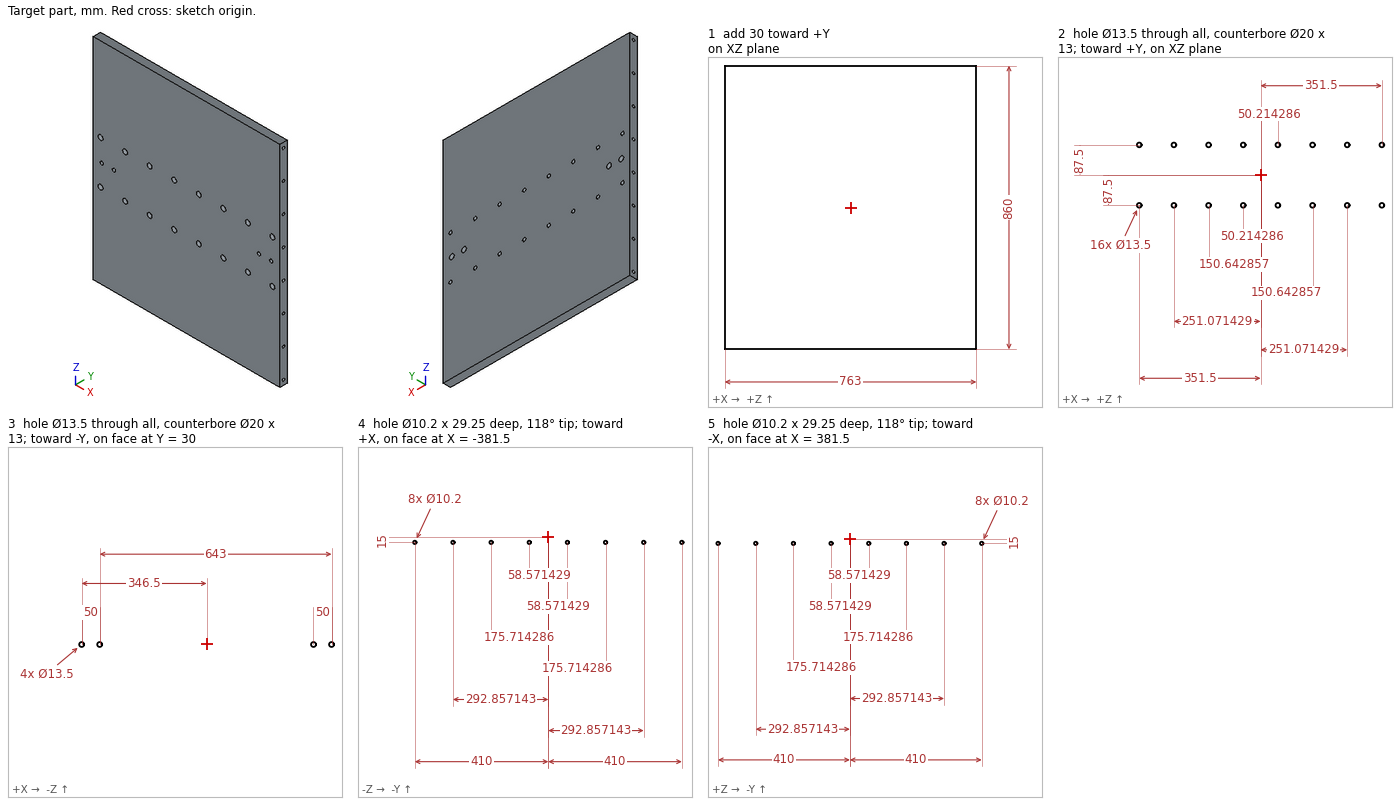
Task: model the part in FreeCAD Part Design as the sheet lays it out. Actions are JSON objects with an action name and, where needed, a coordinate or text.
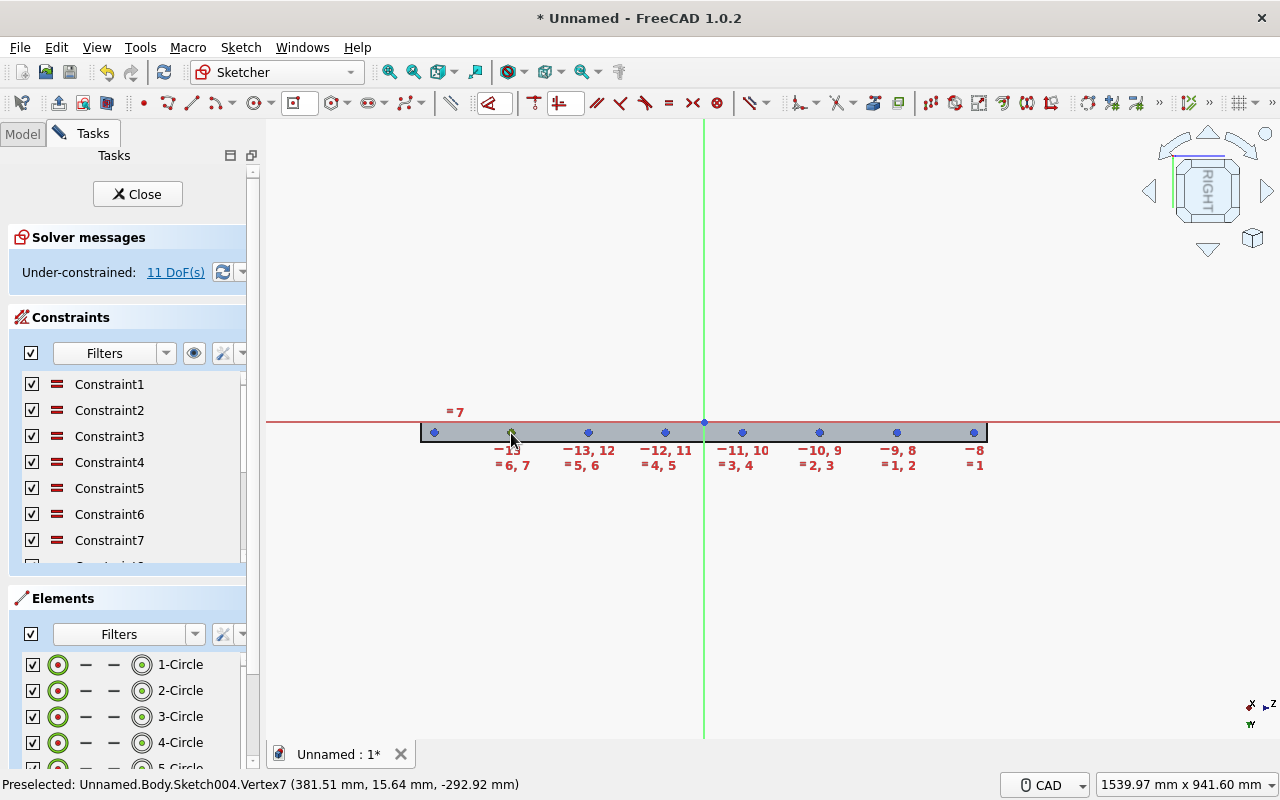
{"action": "left_click", "coordinate": [434, 433]}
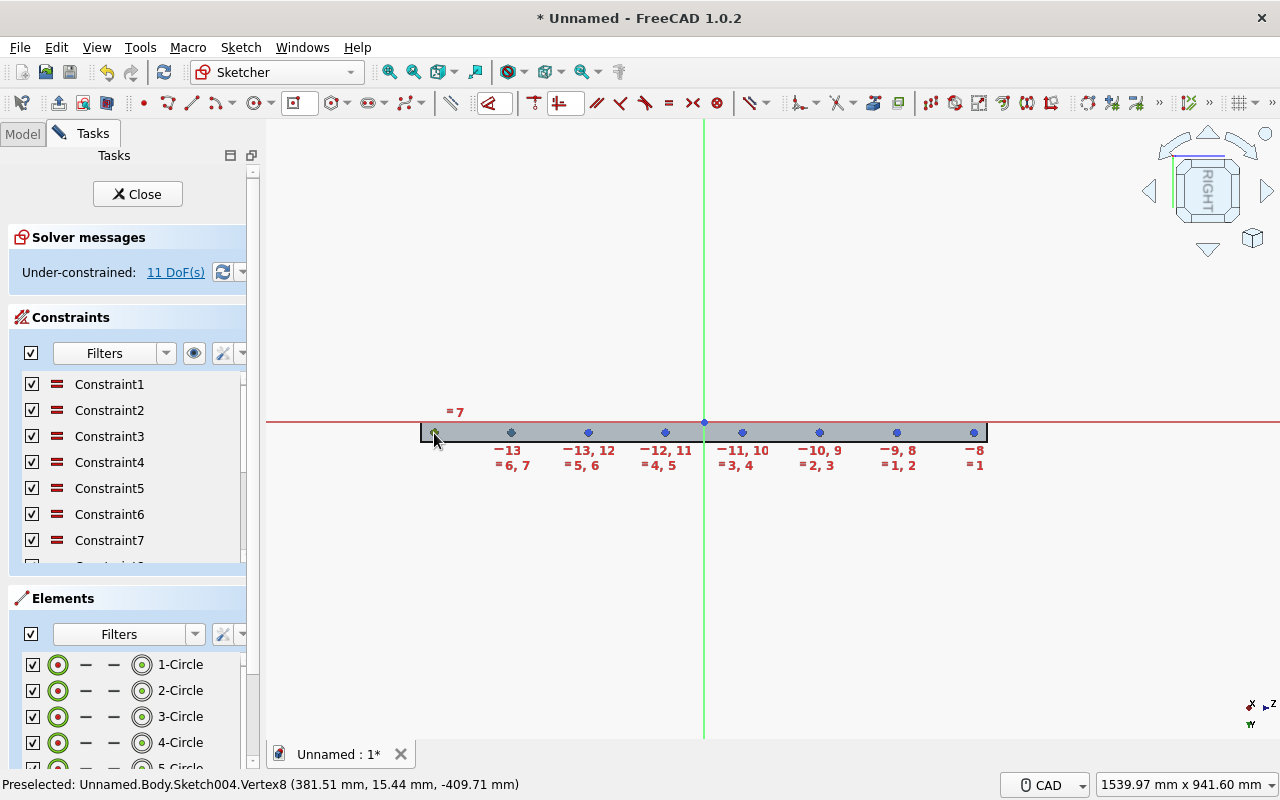
{"action": "key", "text": "h"}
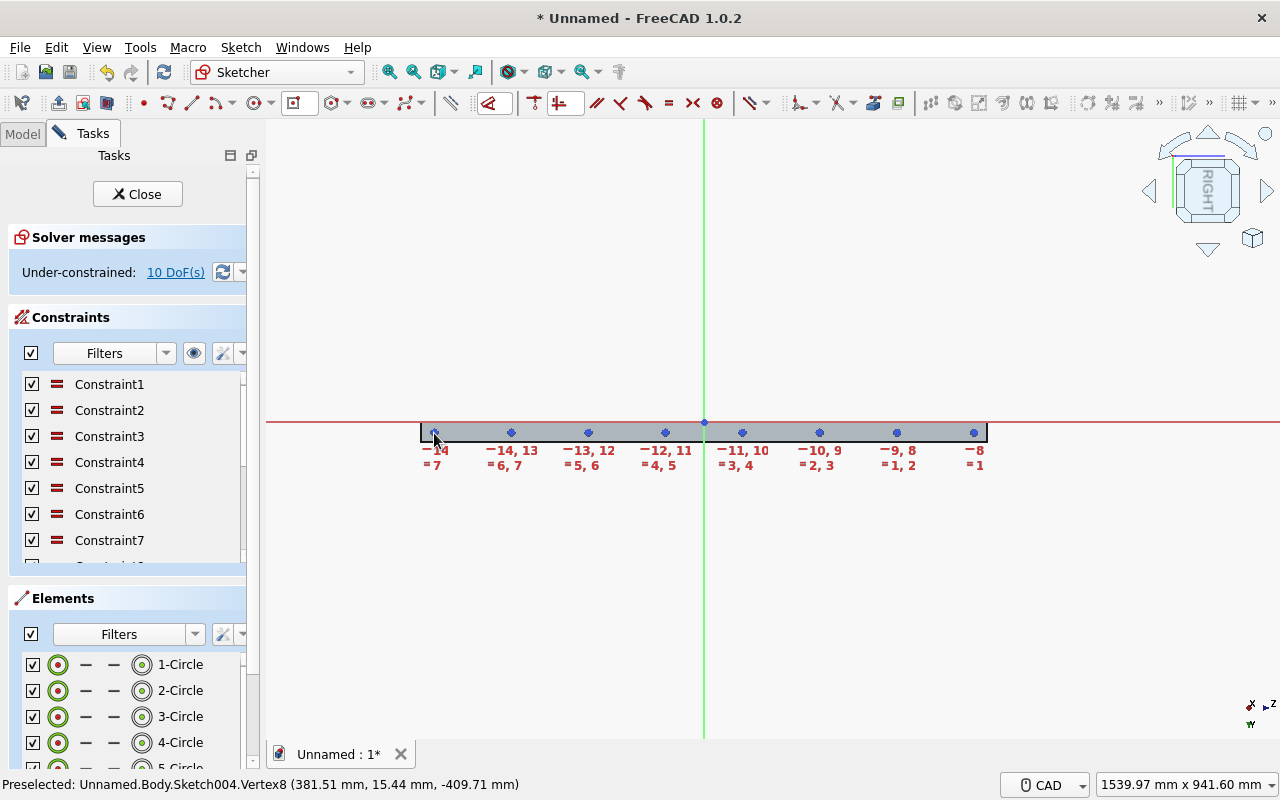
{"action": "scroll", "coordinate": [976, 435], "scroll_direction": "up", "scroll_amount": 9}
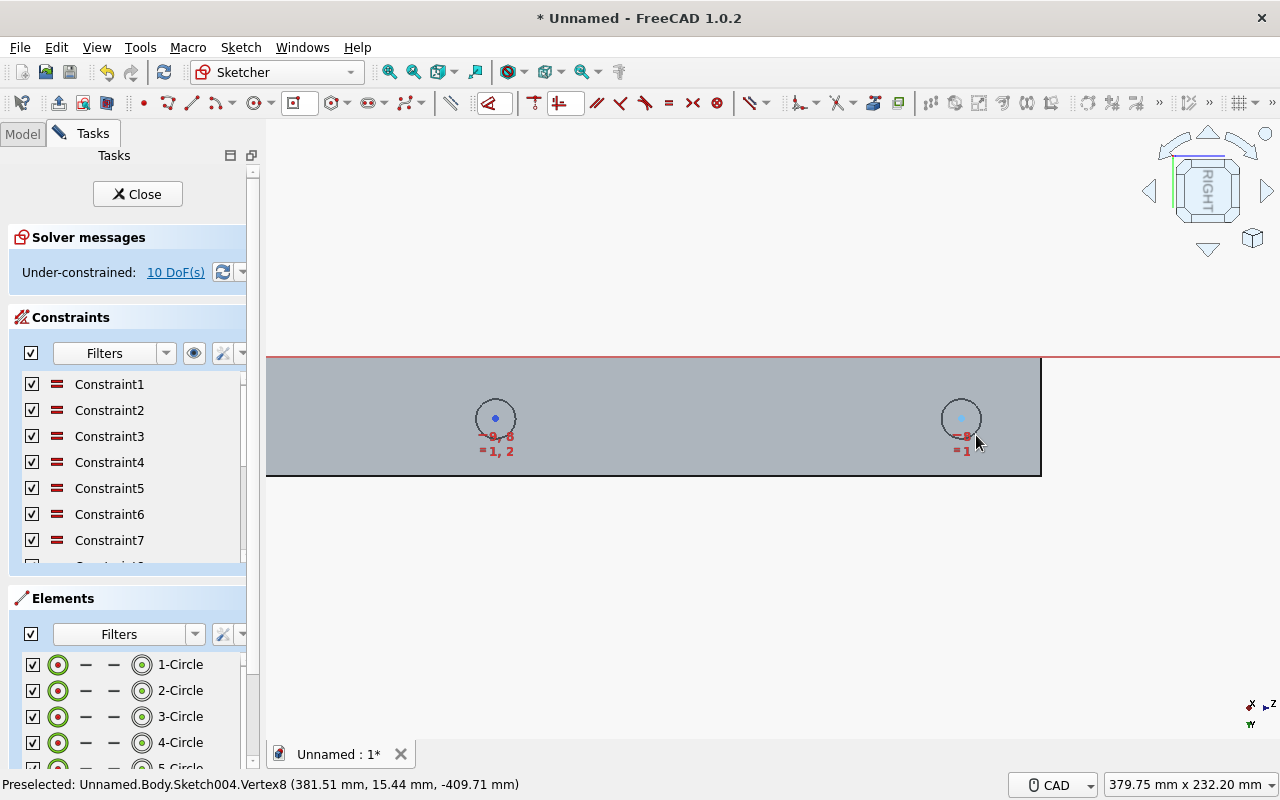
{"action": "left_click", "coordinate": [975, 433]}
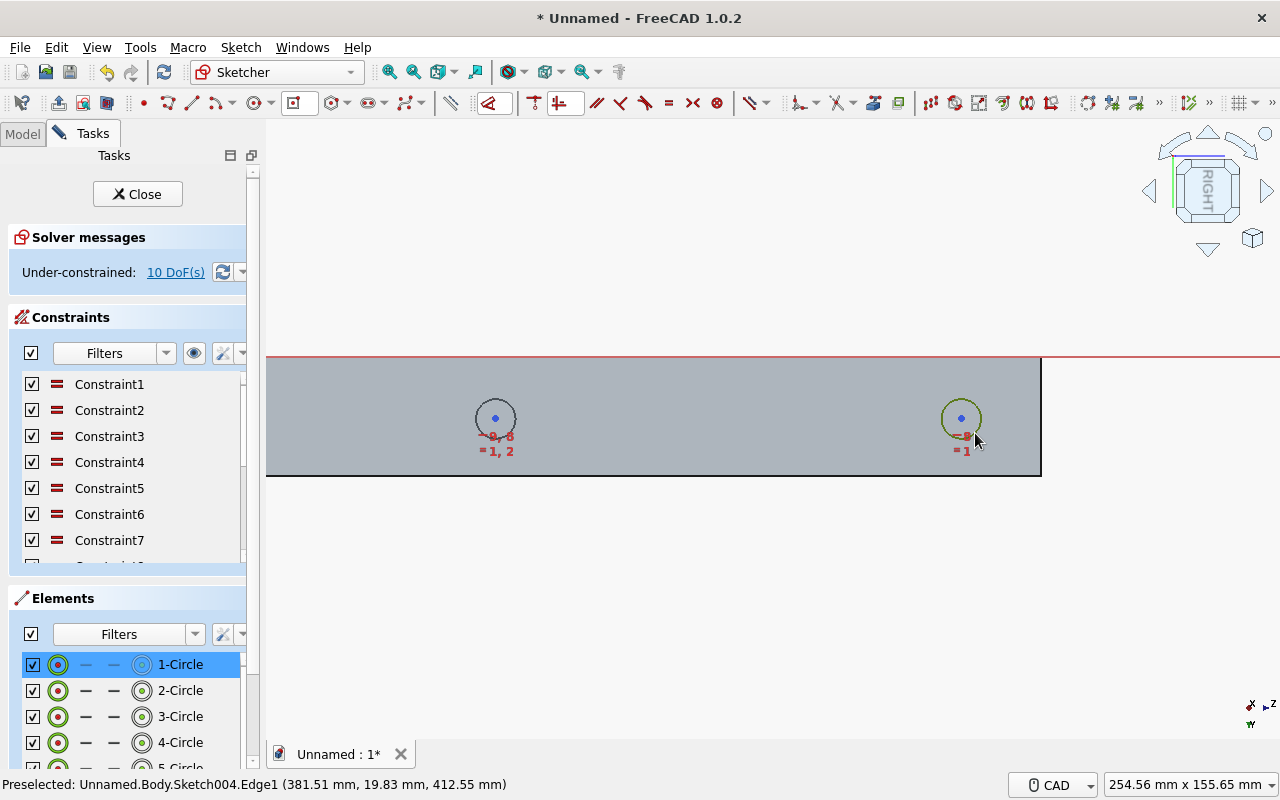
{"action": "key", "text": "k o"}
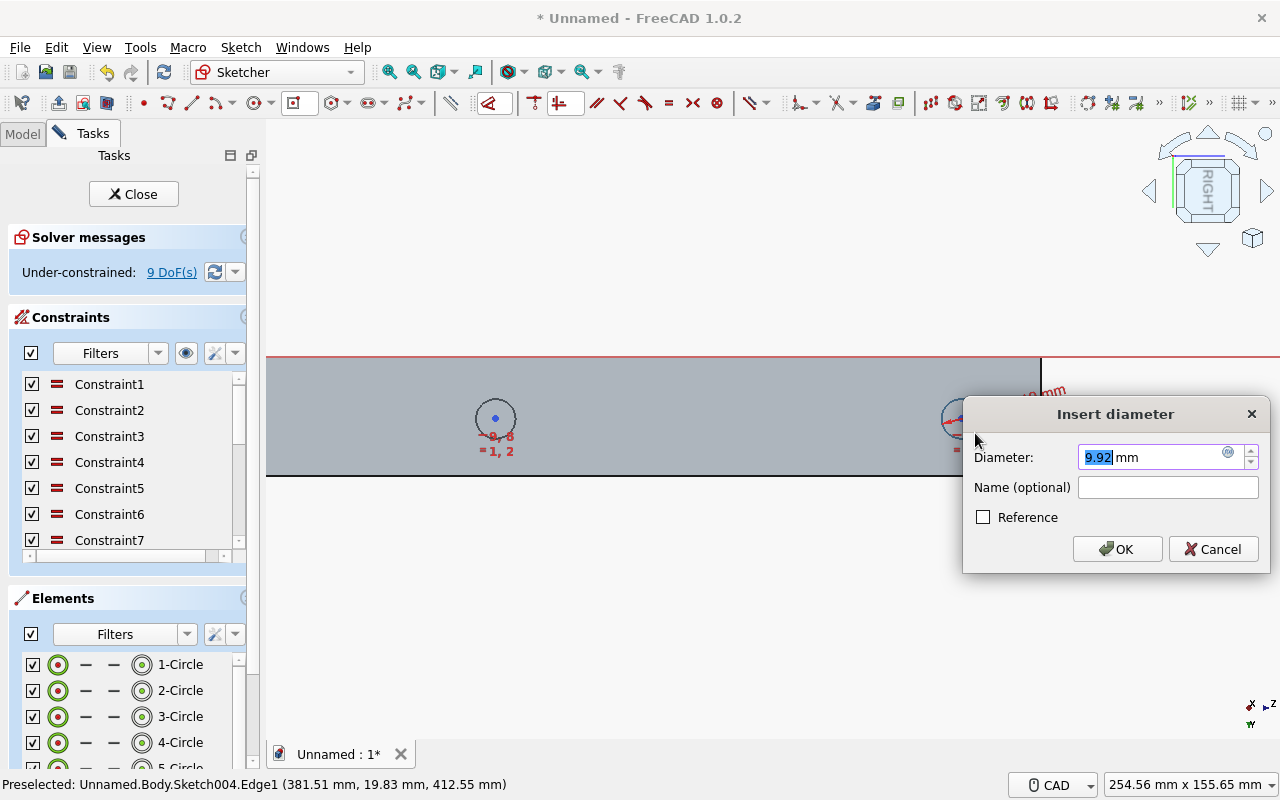
{"action": "type", "text": "10.2"}
{"action": "key", "text": "Return"}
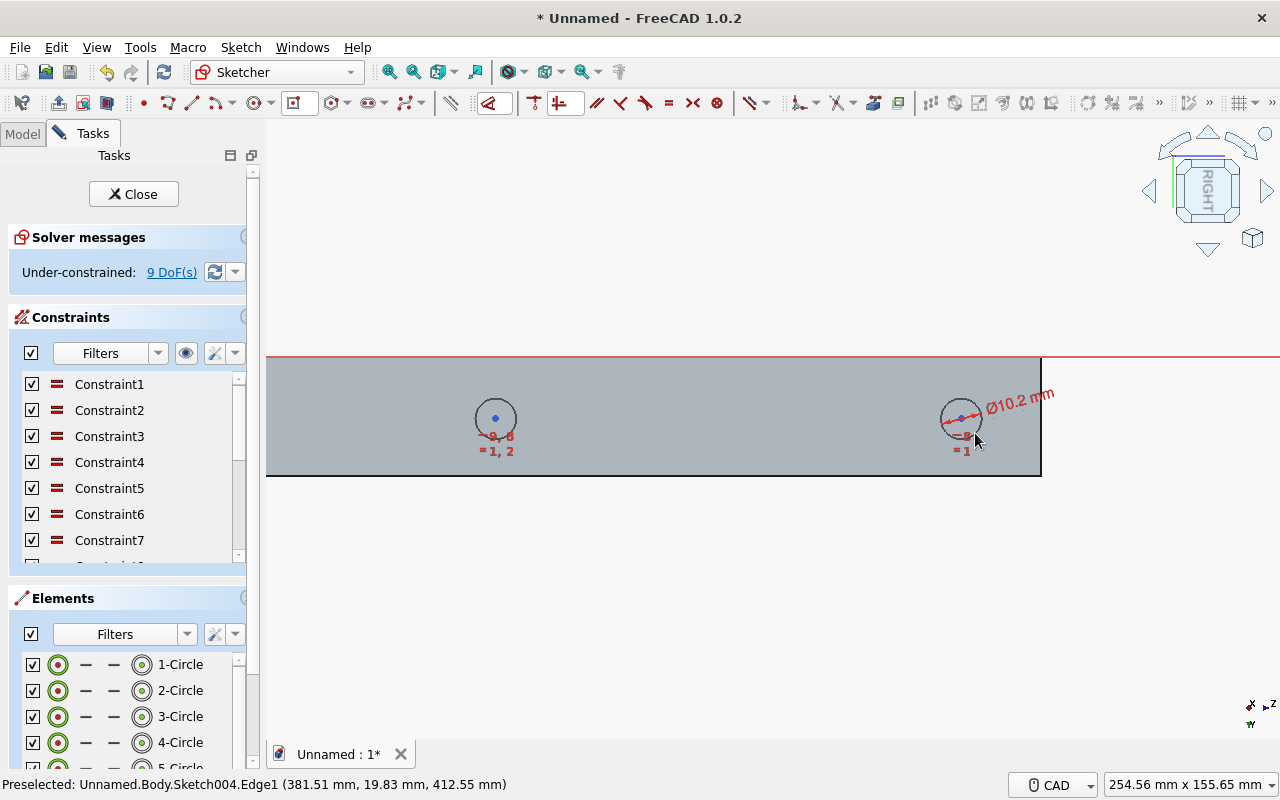
{"action": "left_click", "coordinate": [961, 419]}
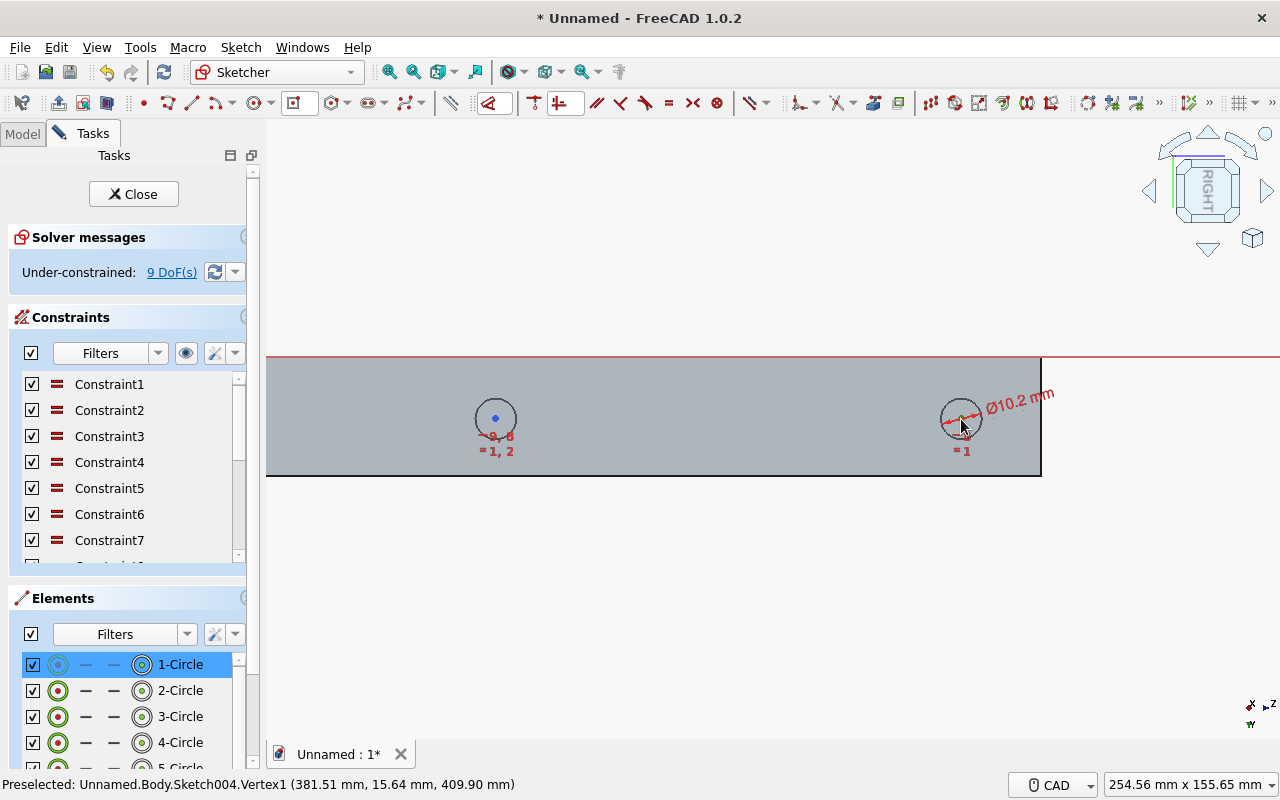
{"action": "key", "text": "i"}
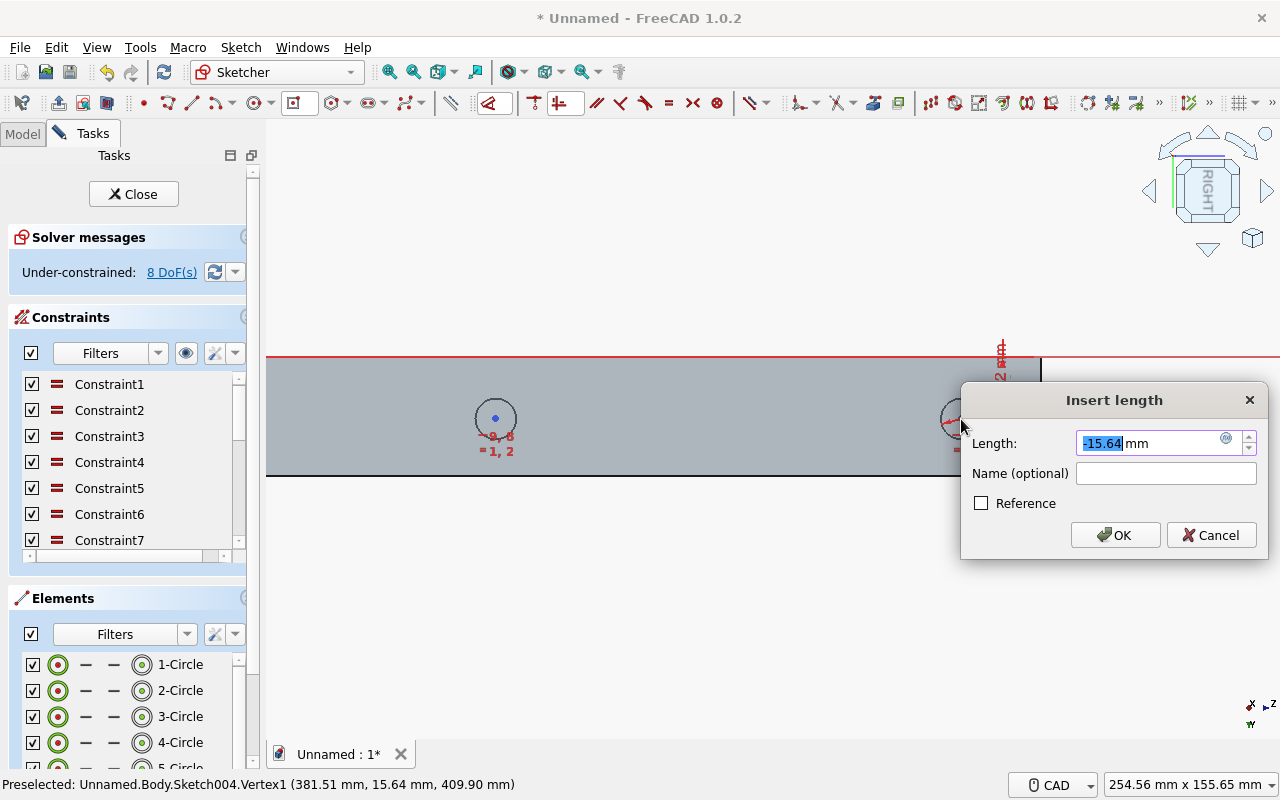
{"action": "type", "text": "-15"}
{"action": "key", "text": "Return"}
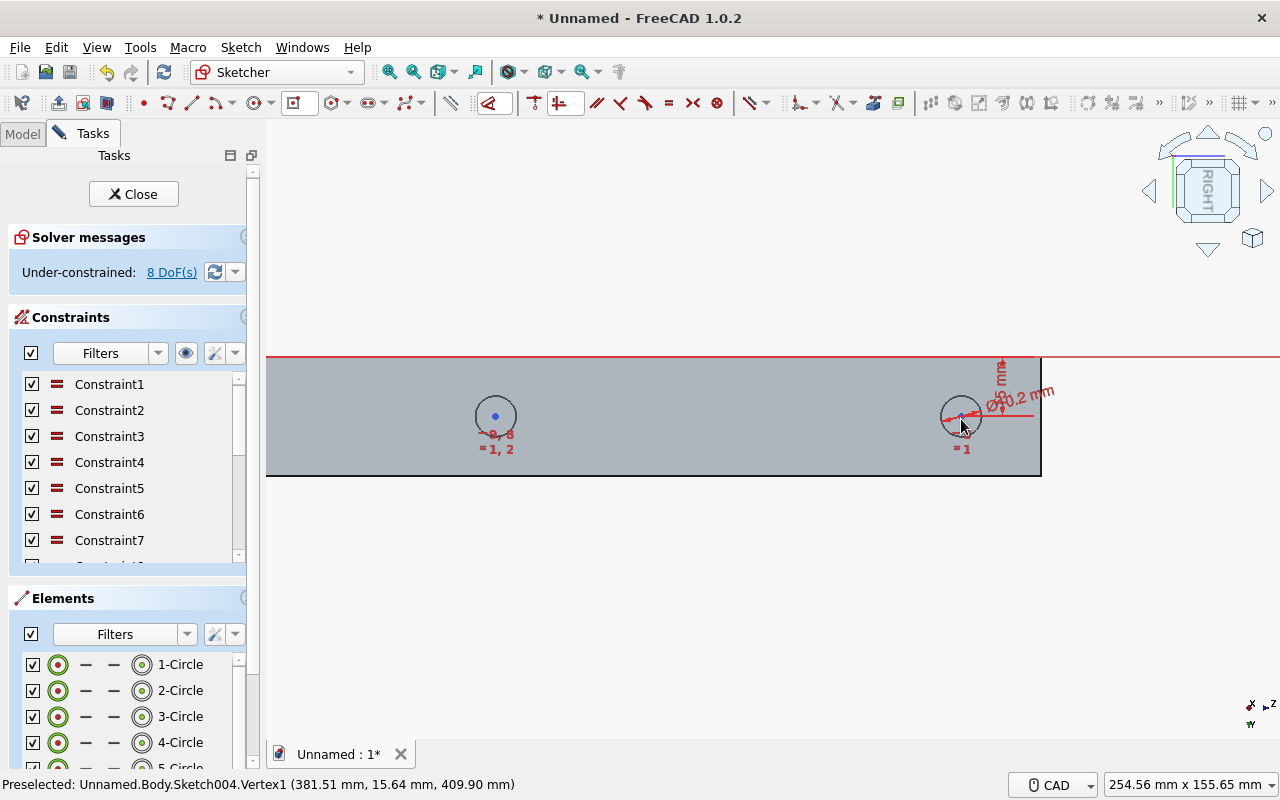
{"action": "scroll", "coordinate": [977, 435], "scroll_direction": "down", "scroll_amount": 9}